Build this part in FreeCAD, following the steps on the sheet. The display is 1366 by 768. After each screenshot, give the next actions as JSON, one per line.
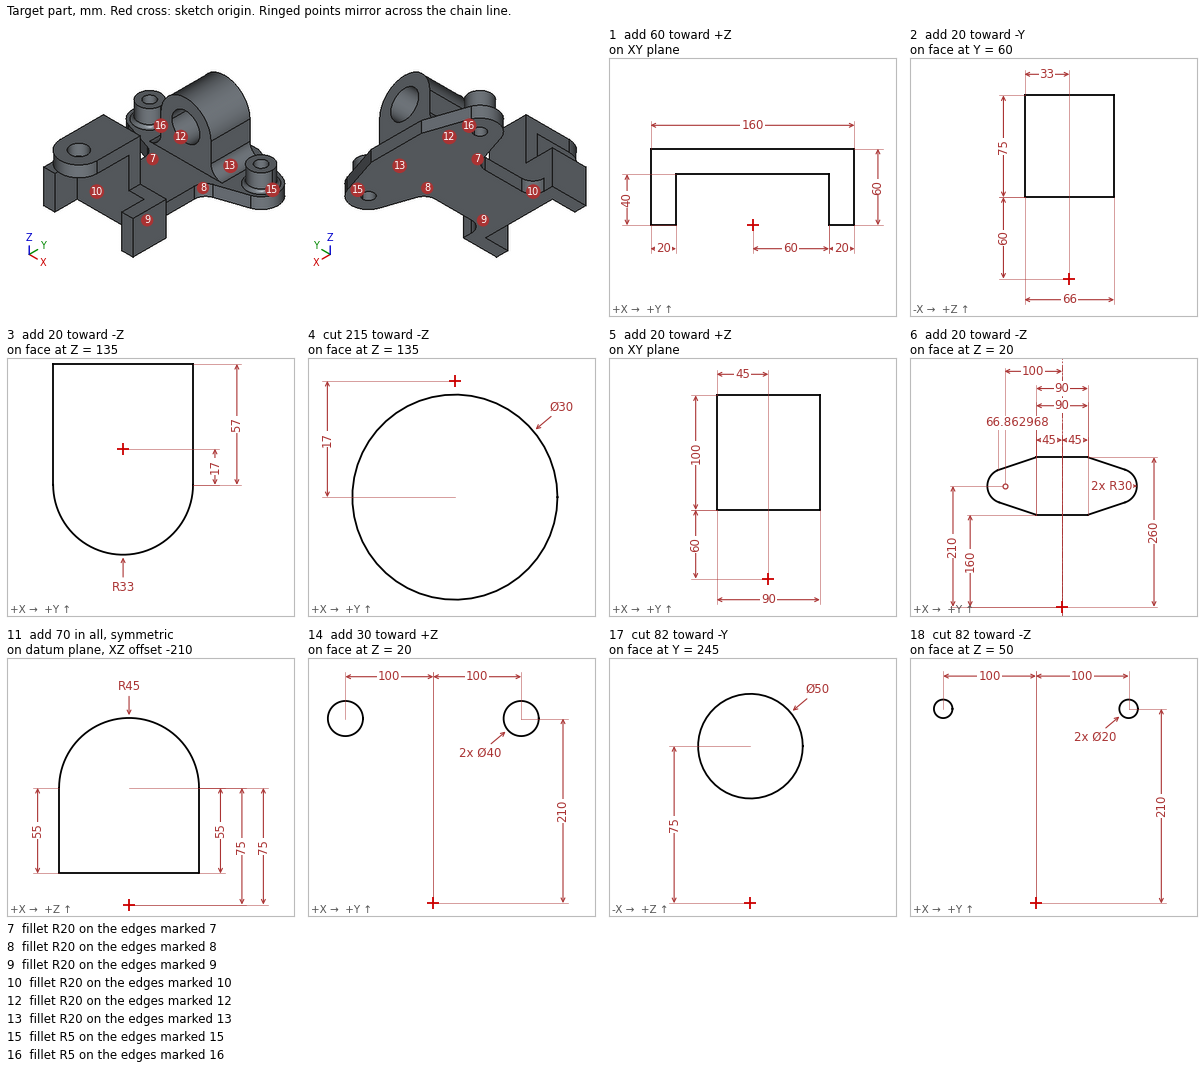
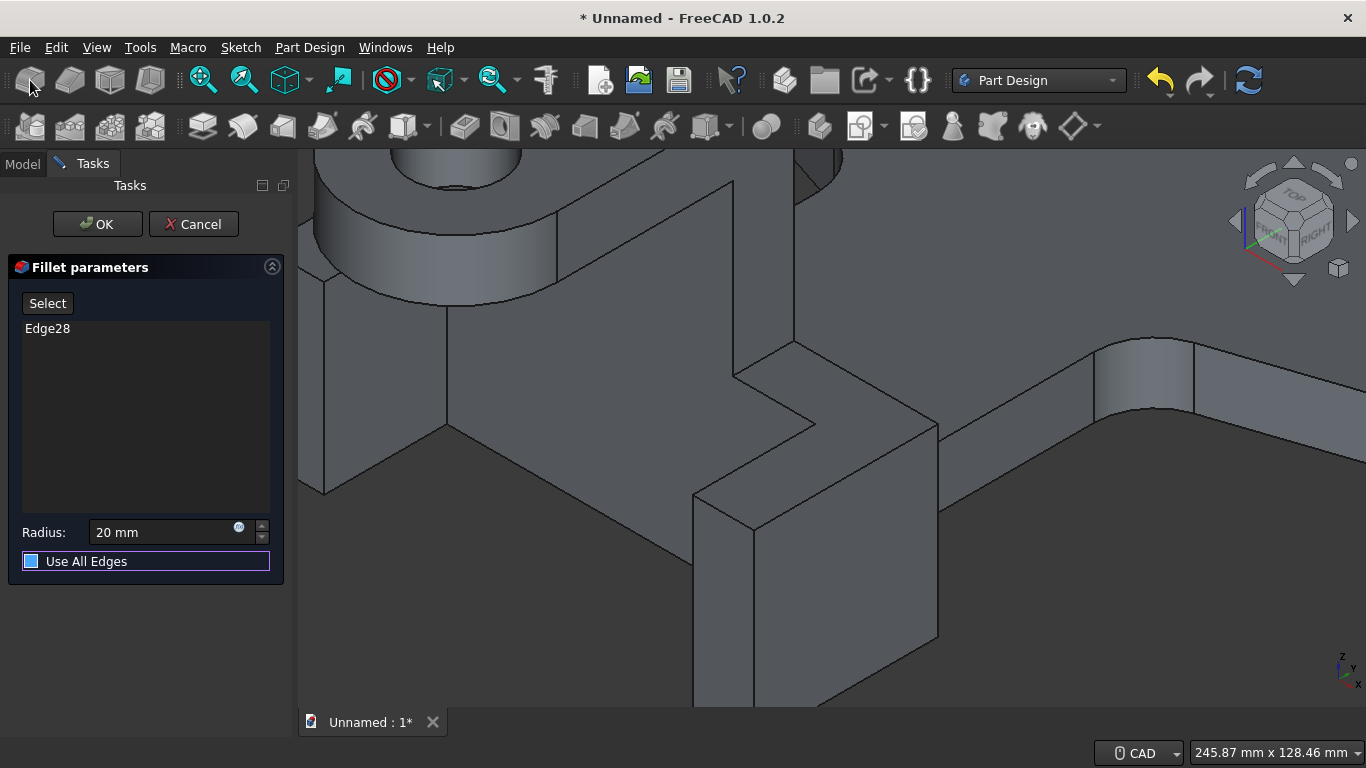
{"action": "left_click", "coordinate": [98, 224]}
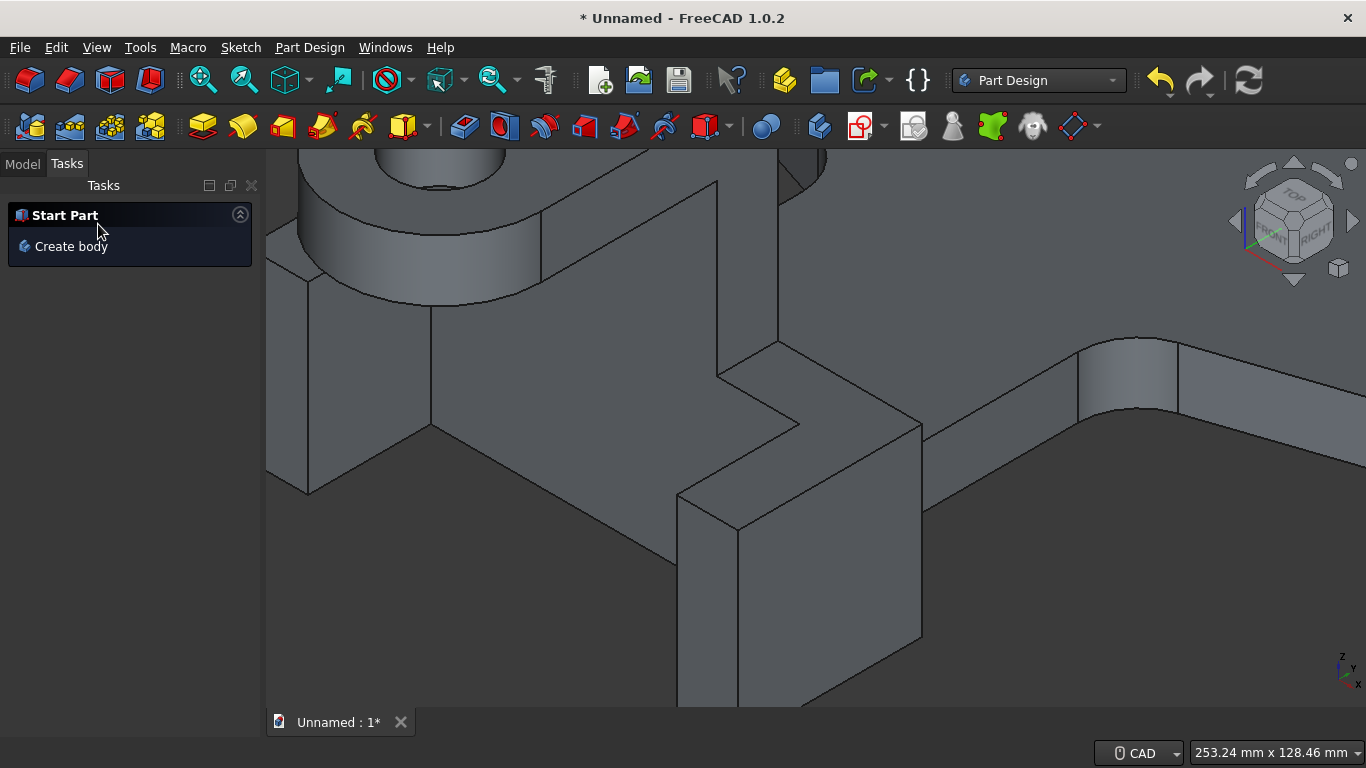
{"action": "key", "text": "v f"}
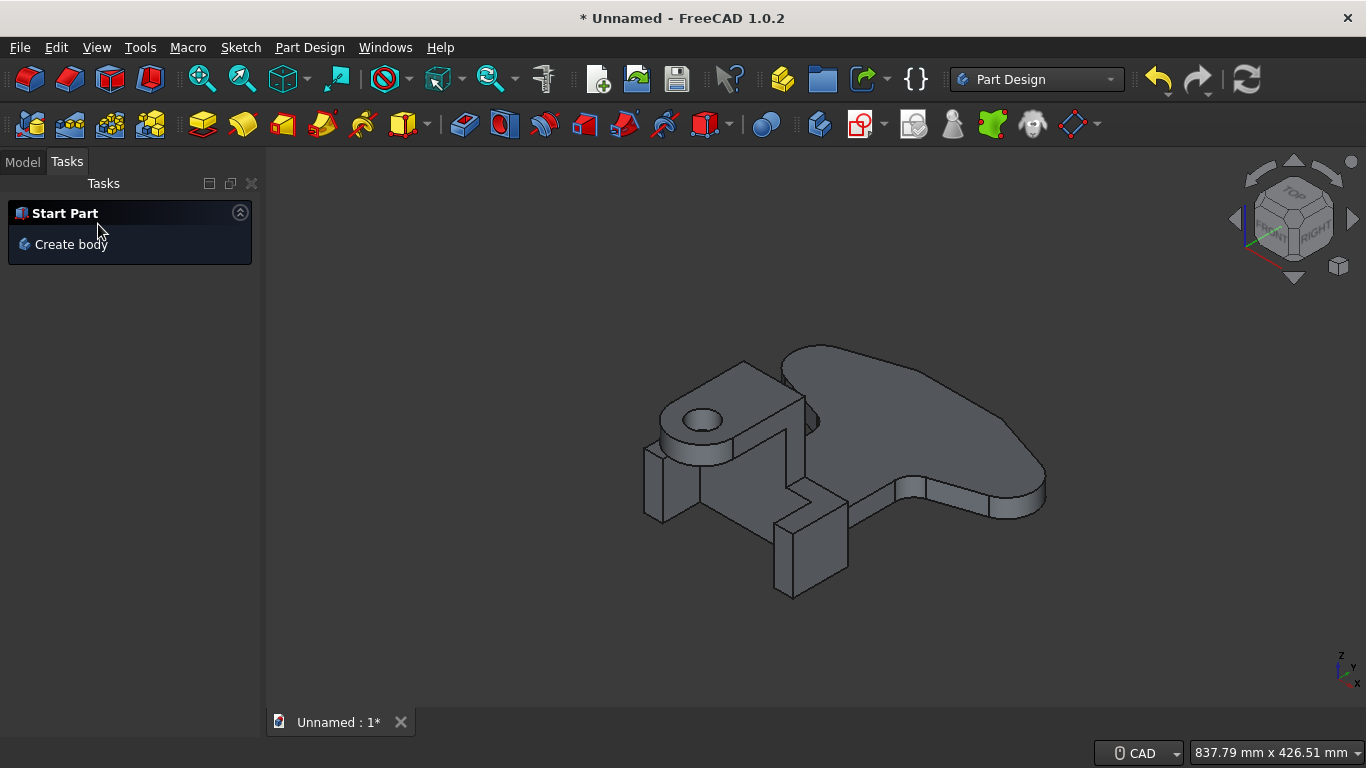
{"action": "key", "text": "2"}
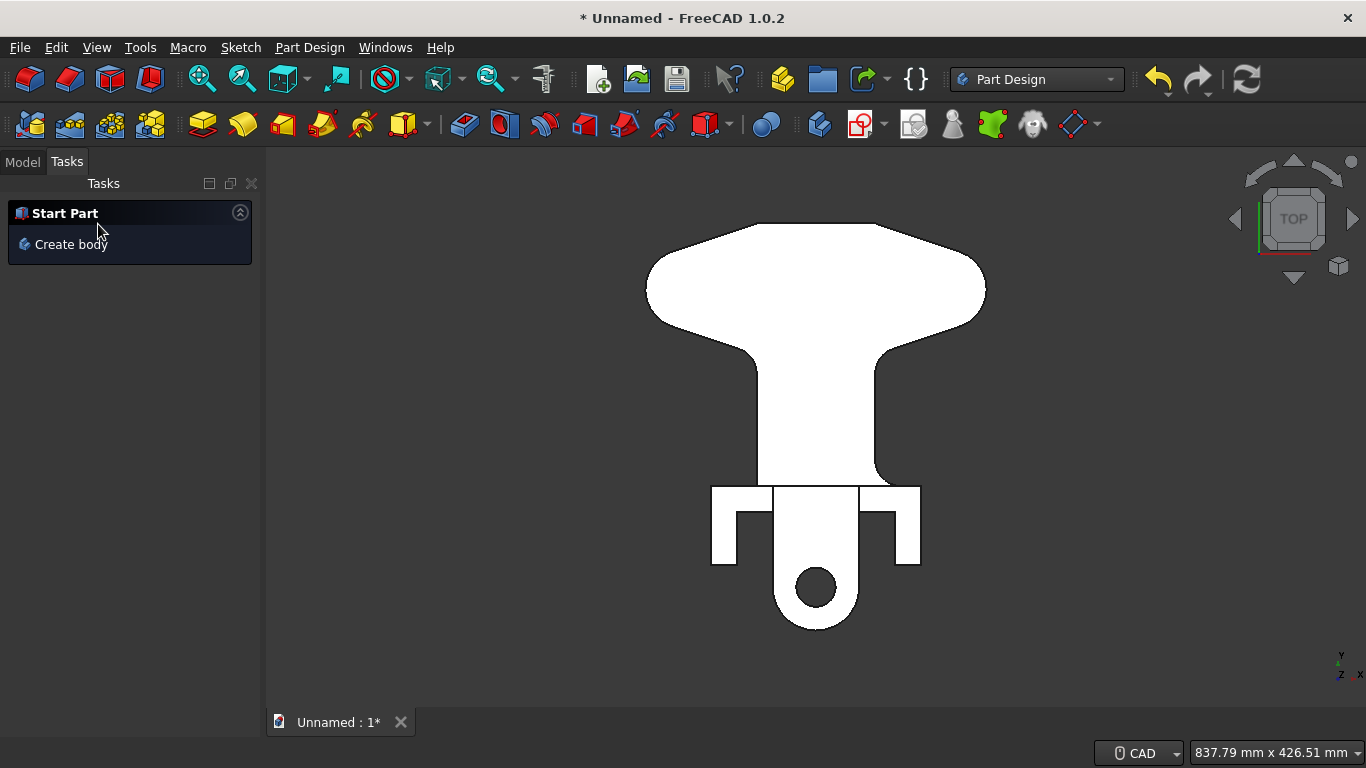
{"action": "key", "text": "0"}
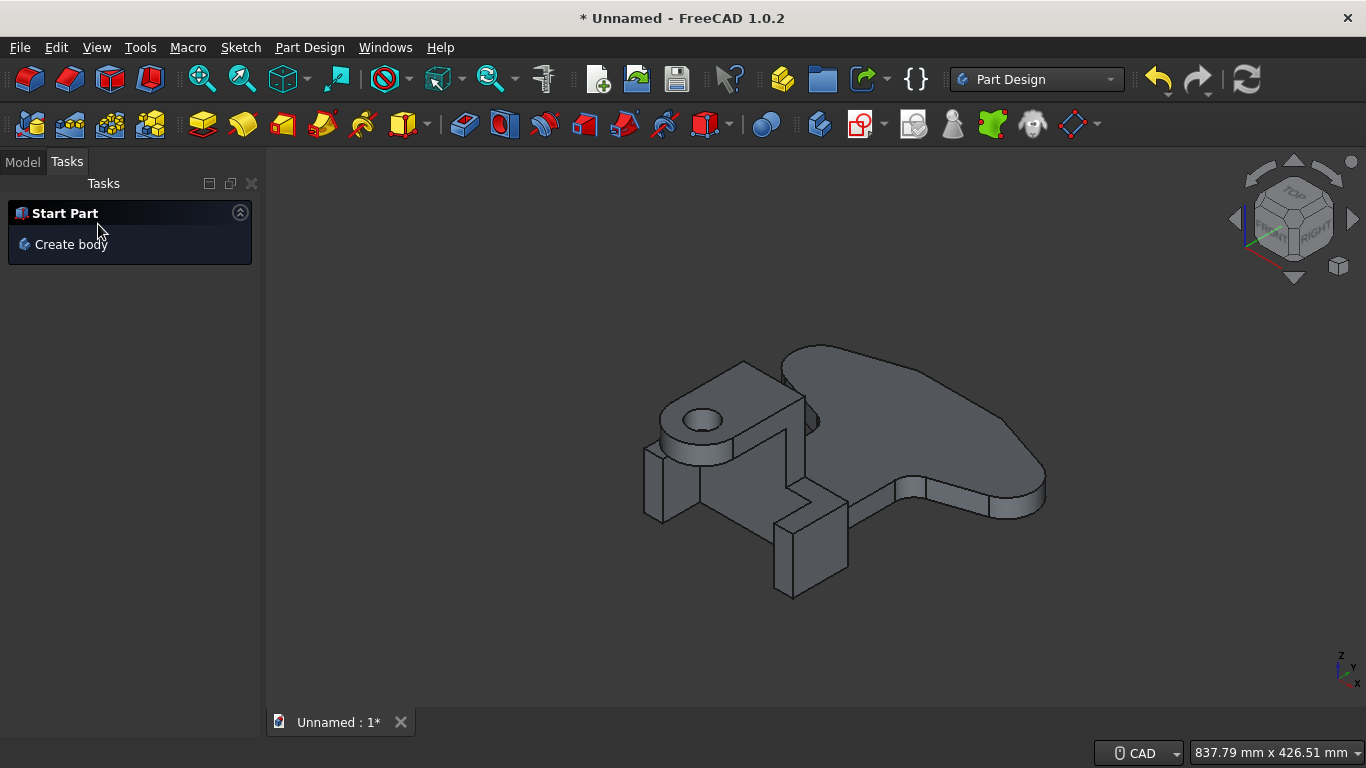
{"action": "key", "text": "1"}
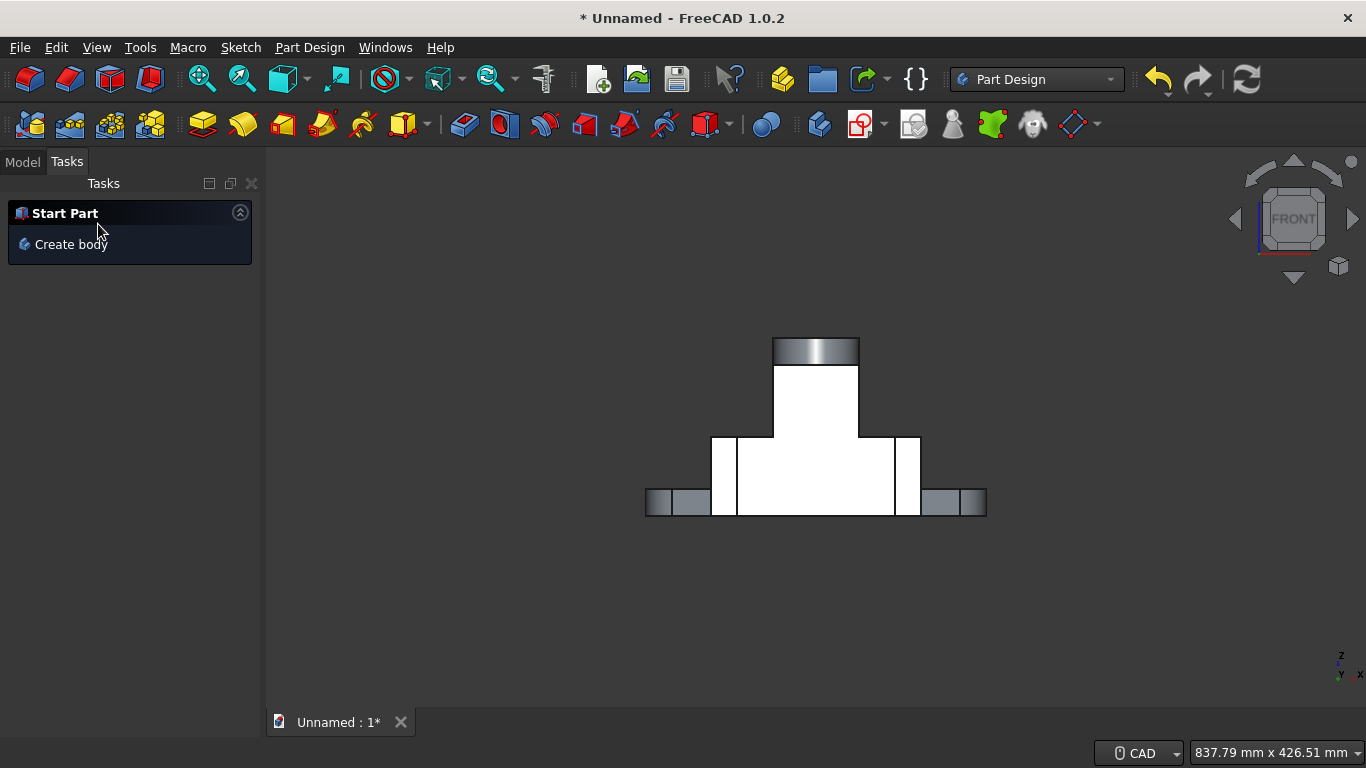
{"action": "left_click", "coordinate": [204, 80]}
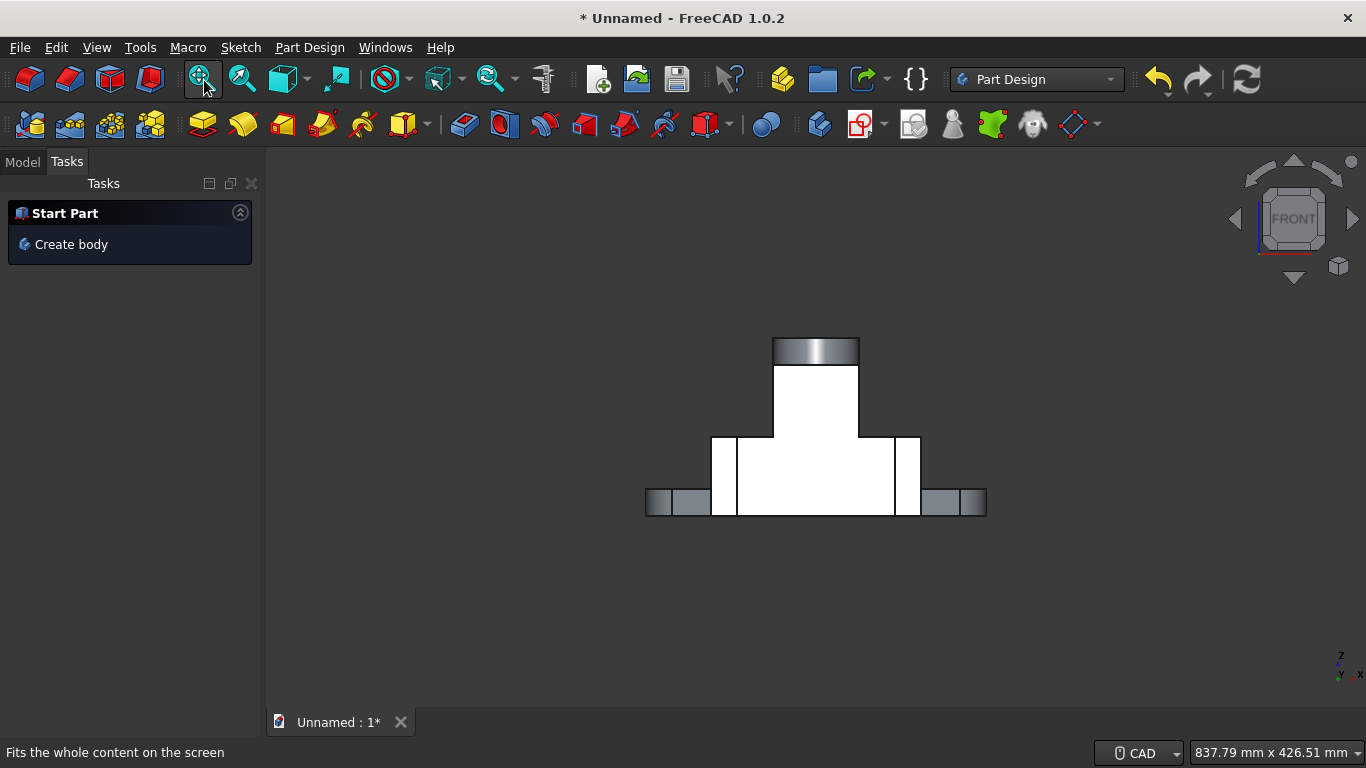
{"action": "key", "text": "3"}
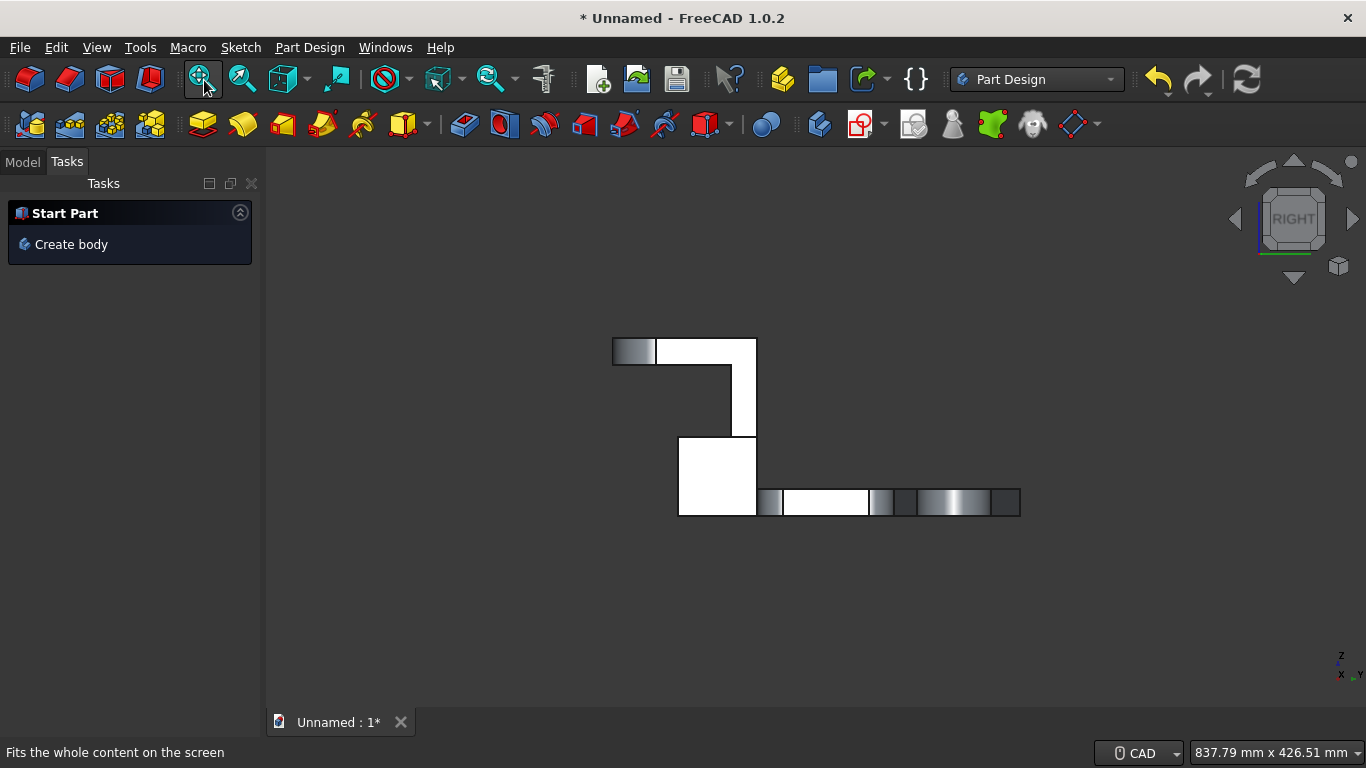
{"action": "key", "text": "v f"}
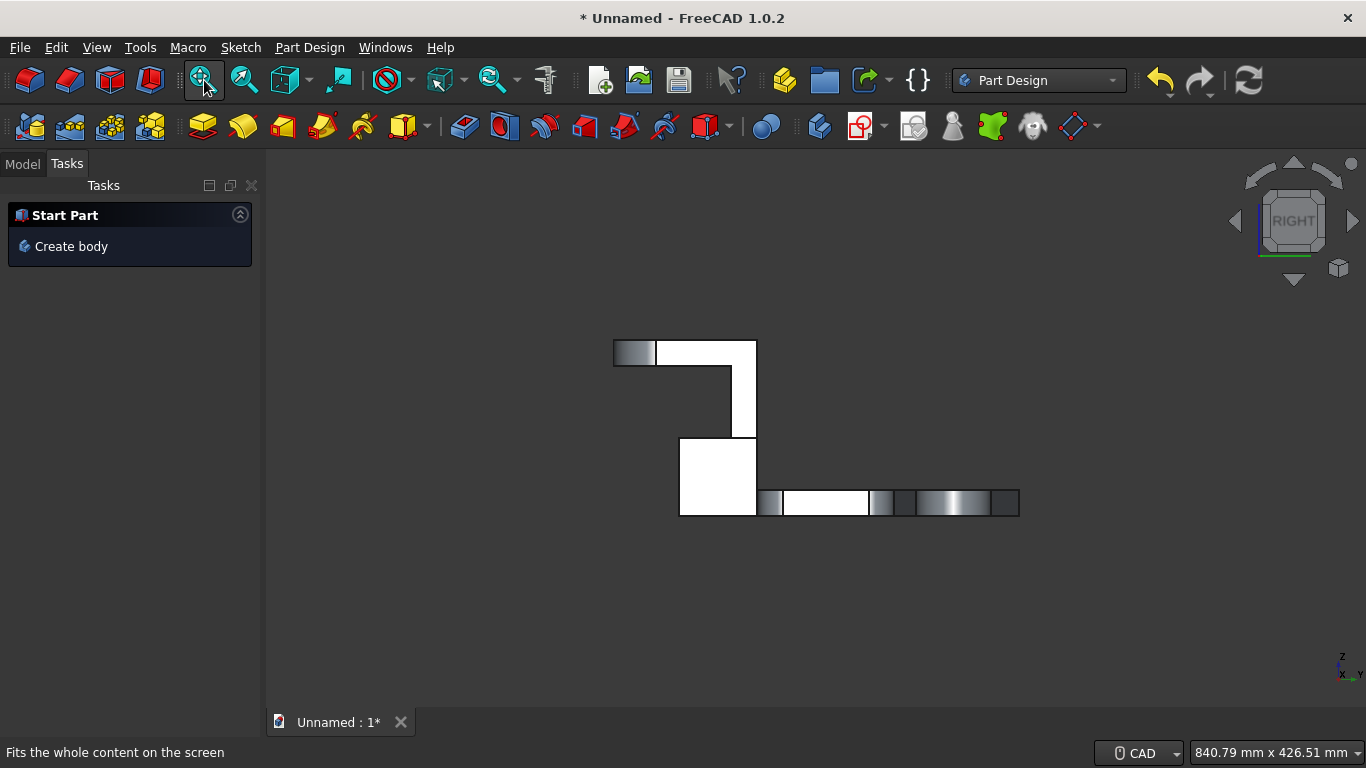
{"action": "key", "text": "5"}